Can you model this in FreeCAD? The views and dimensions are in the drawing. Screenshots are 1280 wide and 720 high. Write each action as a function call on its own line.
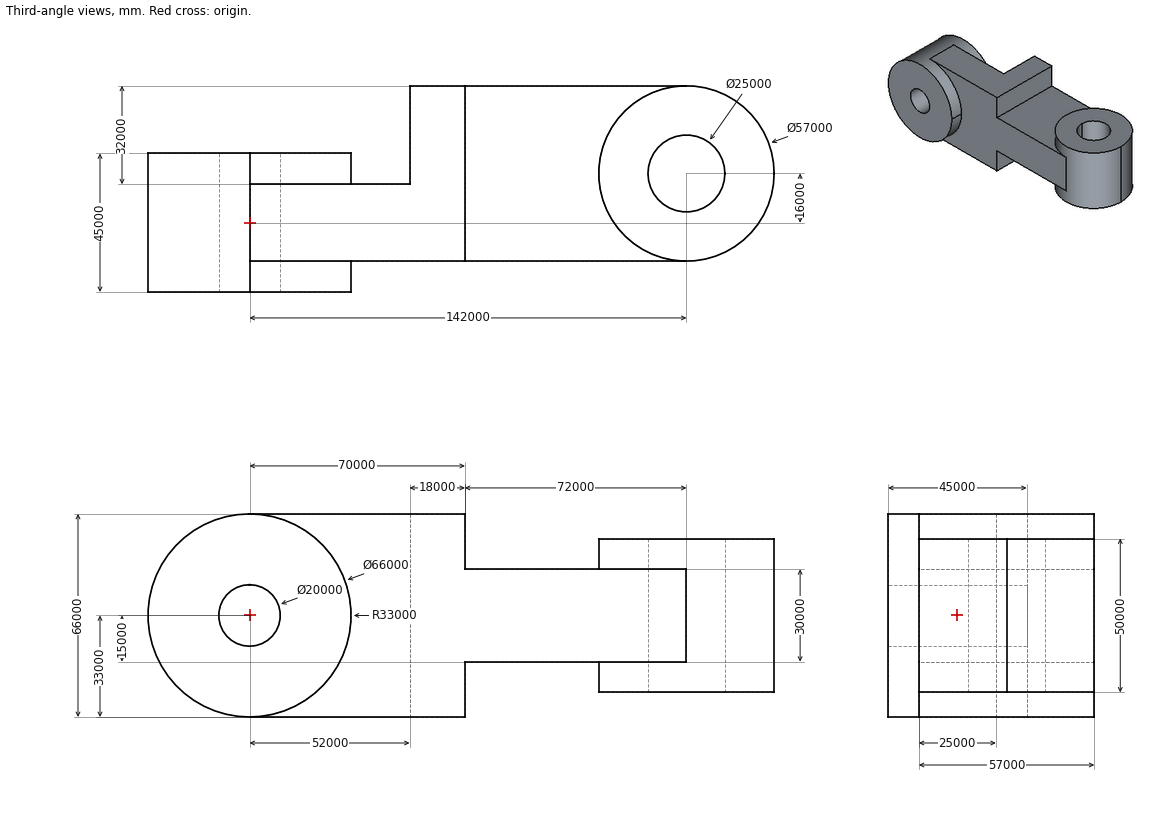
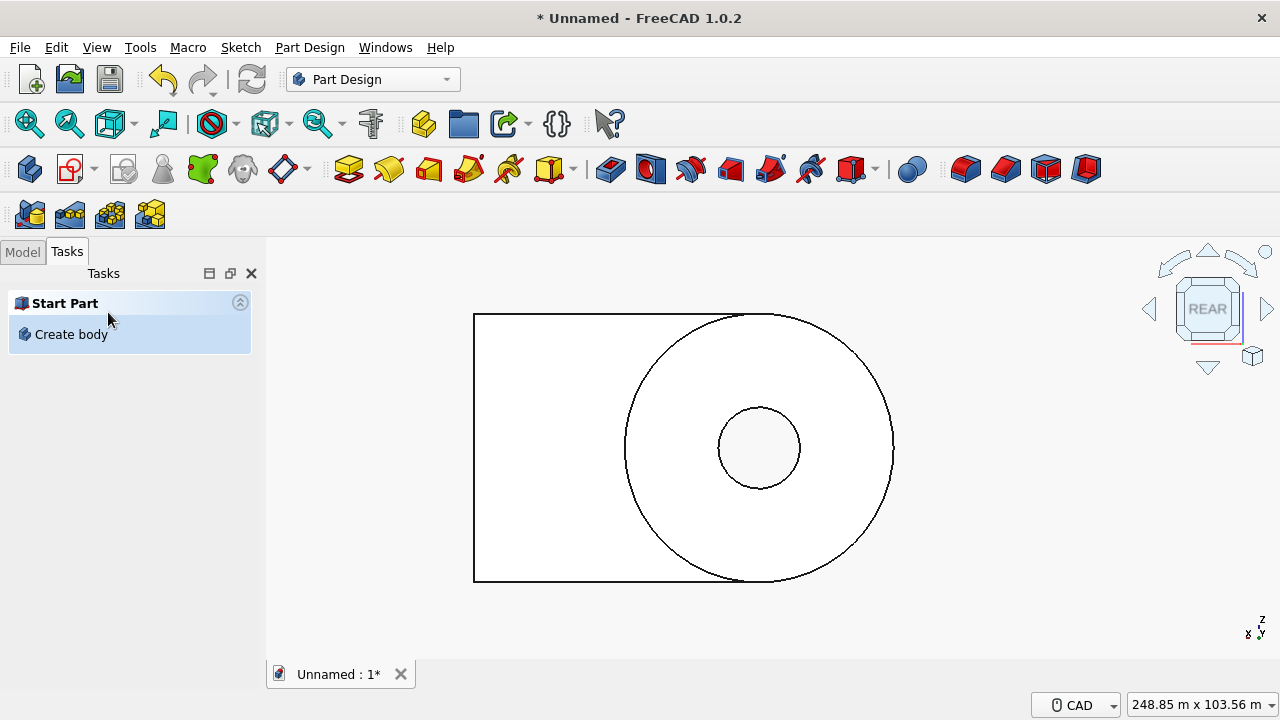
click(535, 409)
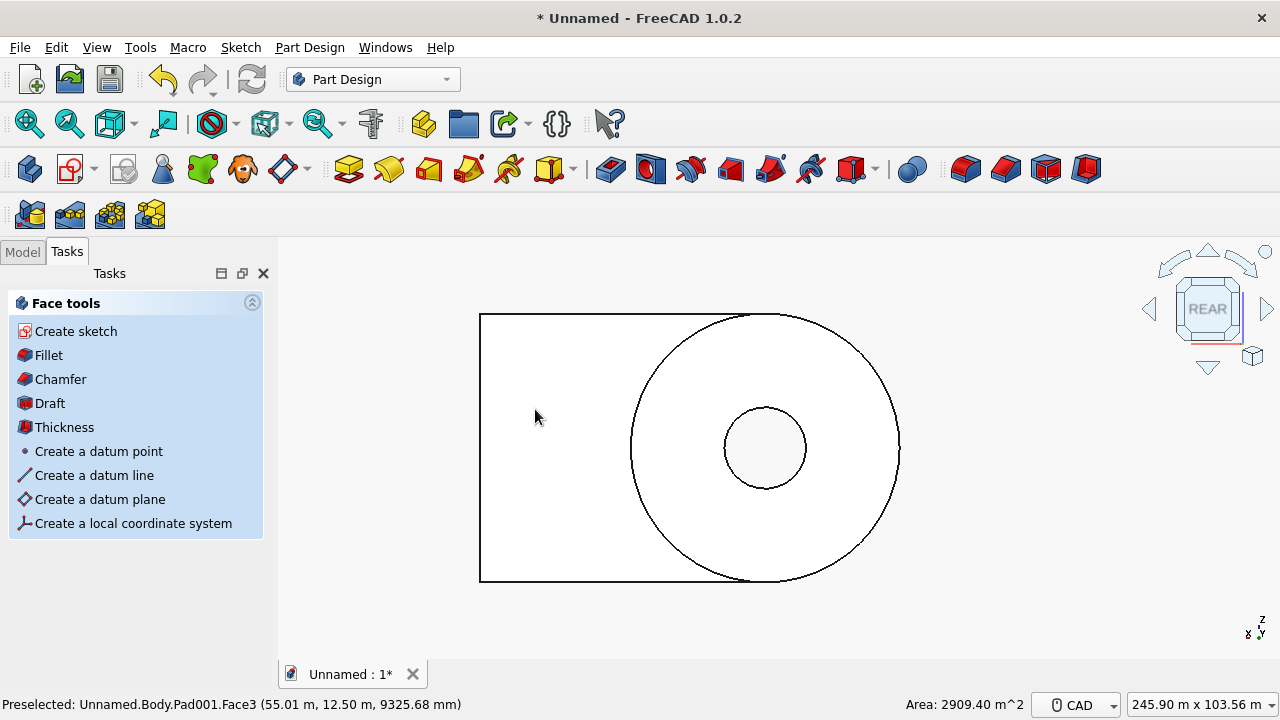
click(70, 170)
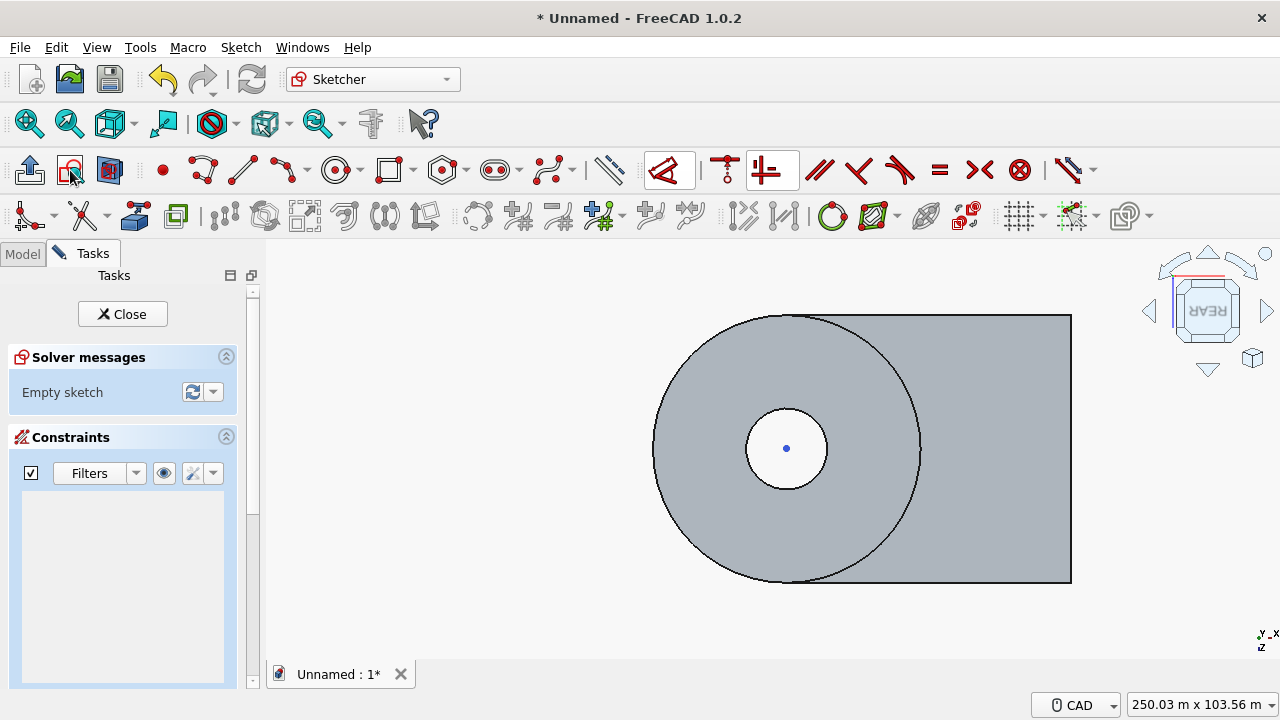
key(q)
key(s)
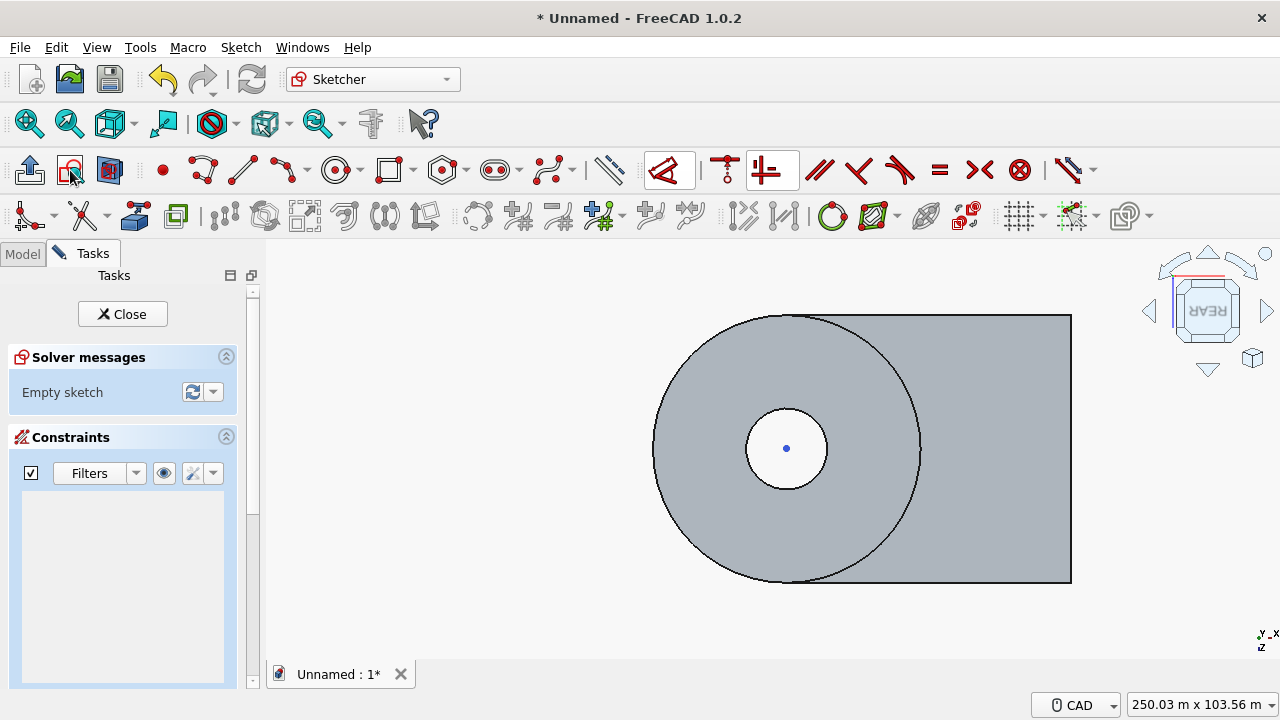
key(g)
key(r)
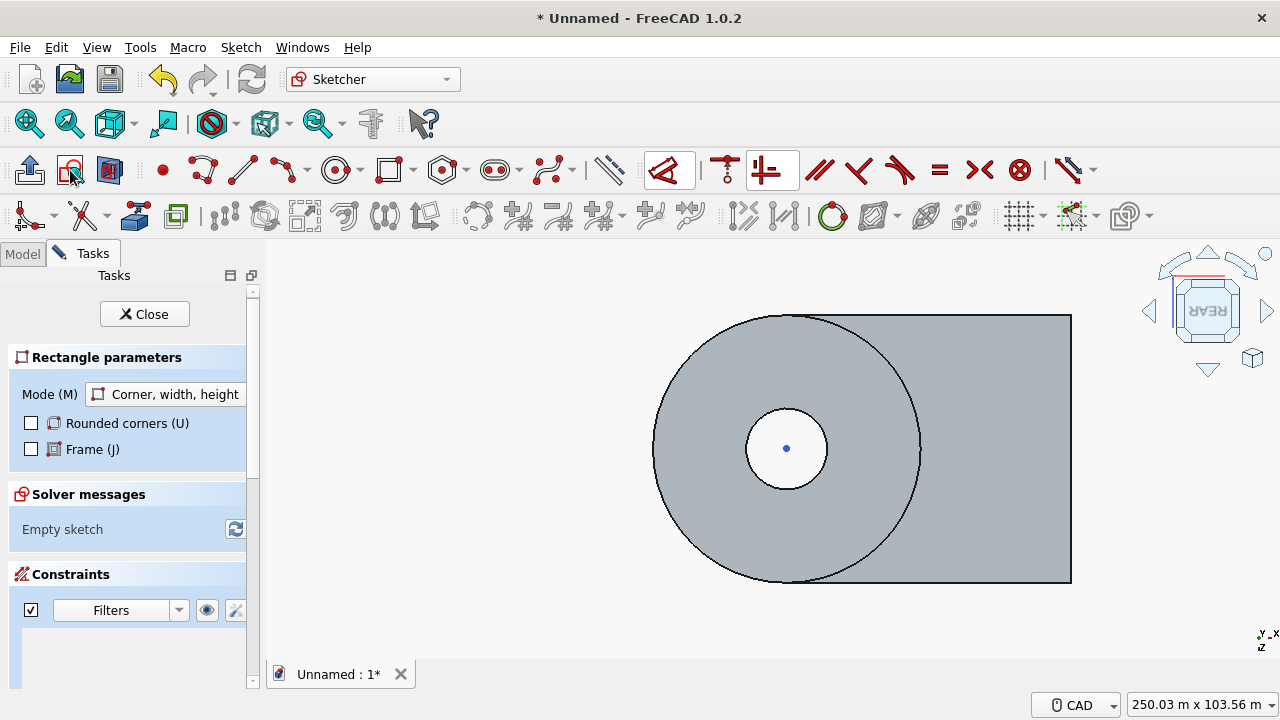
click(998, 315)
click(1071, 583)
key(Escape)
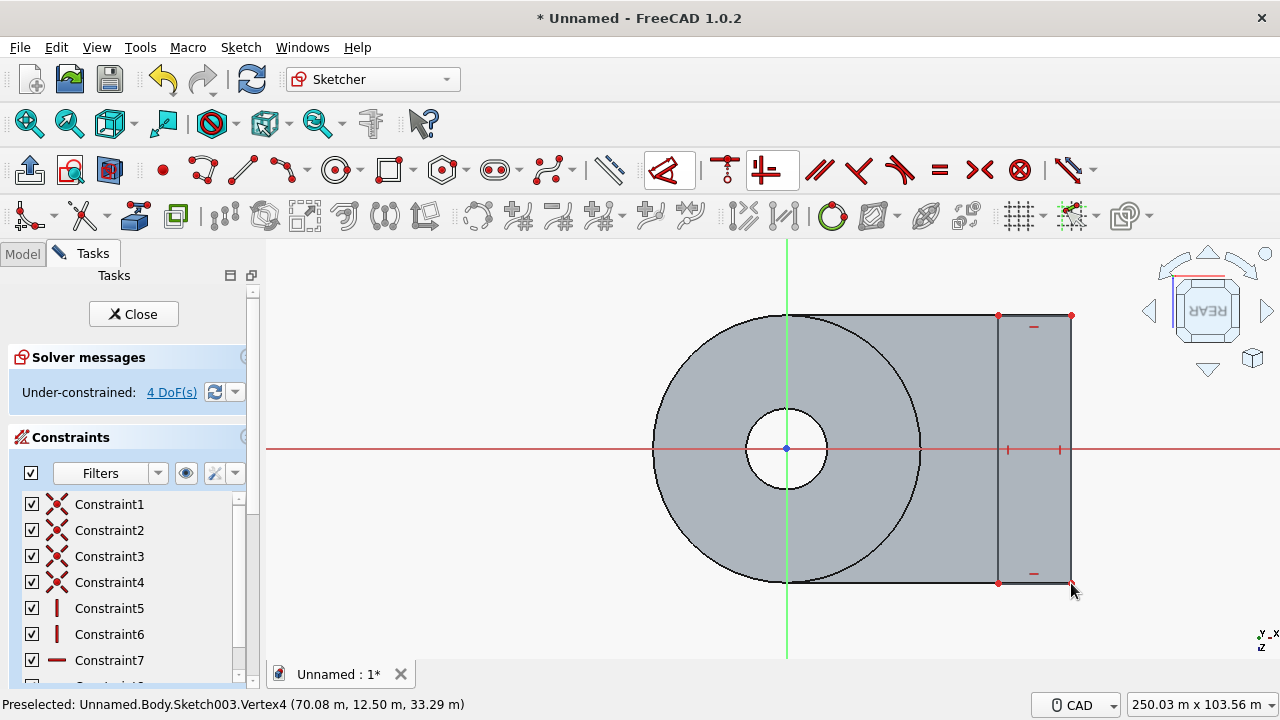
key(d)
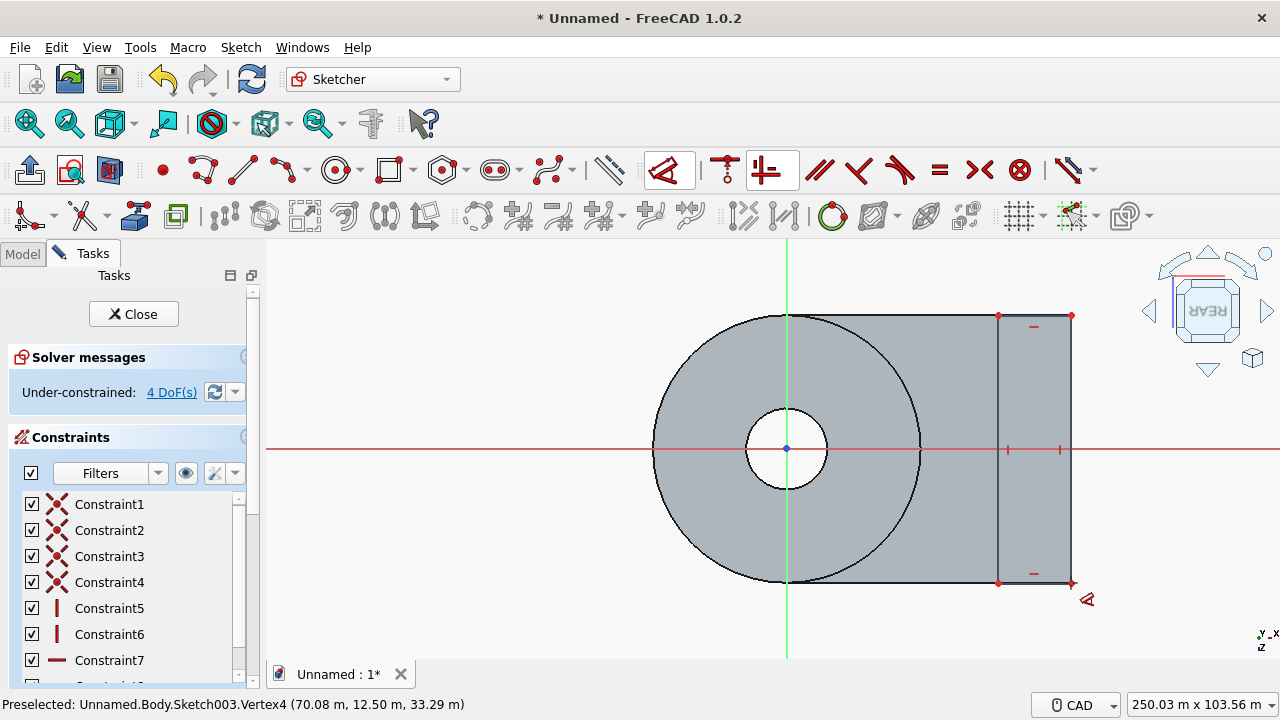
click(998, 396)
click(1032, 388)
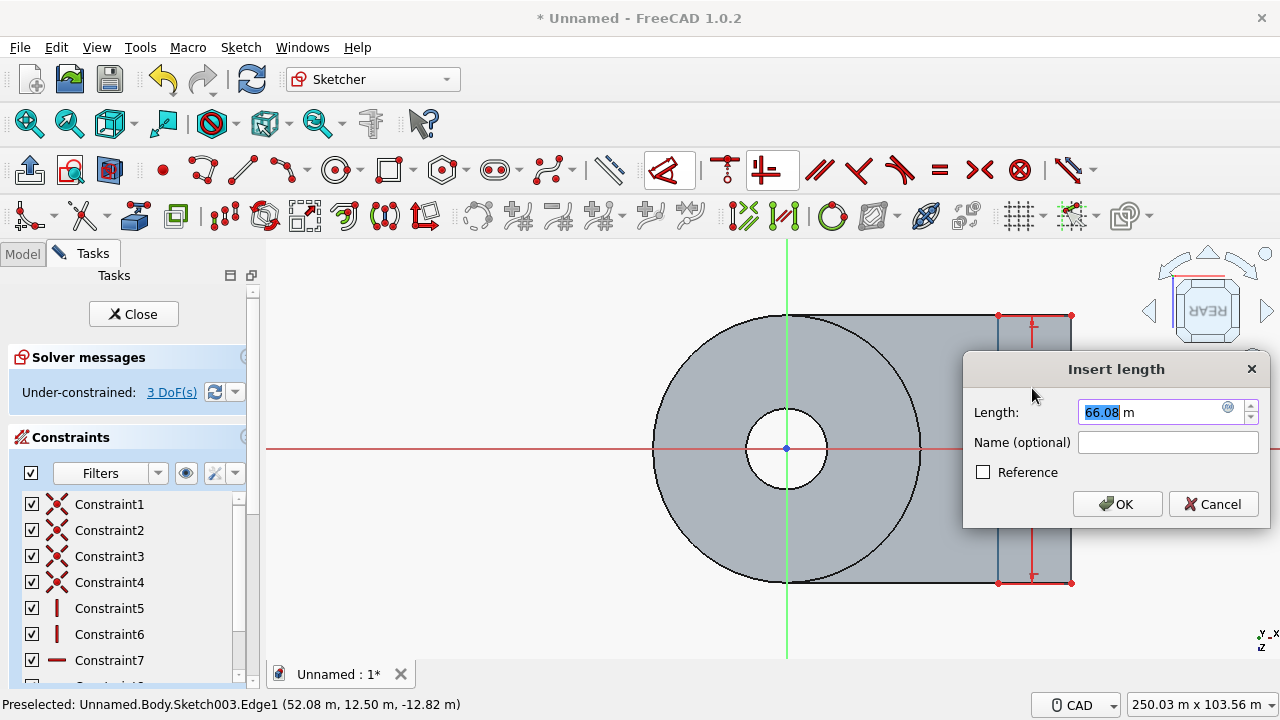
key(ctrl+a)
text(66000 mm)
key(Return)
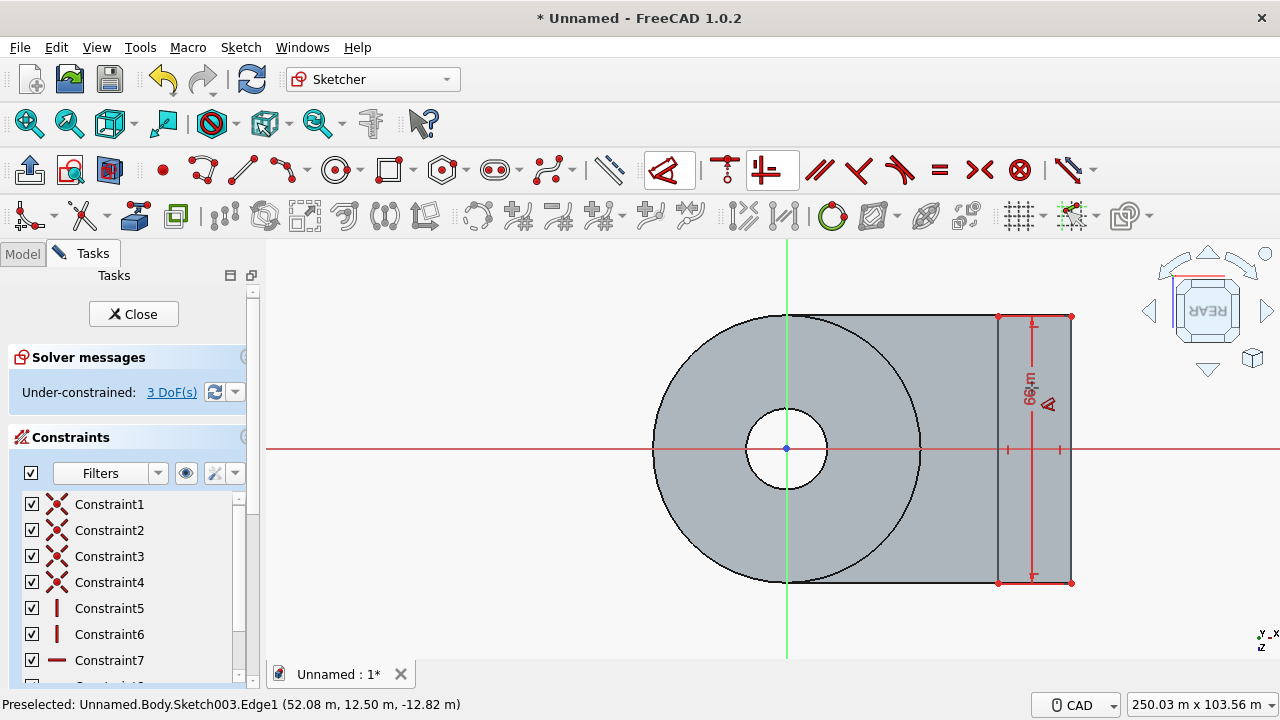
click(1020, 584)
click(1034, 618)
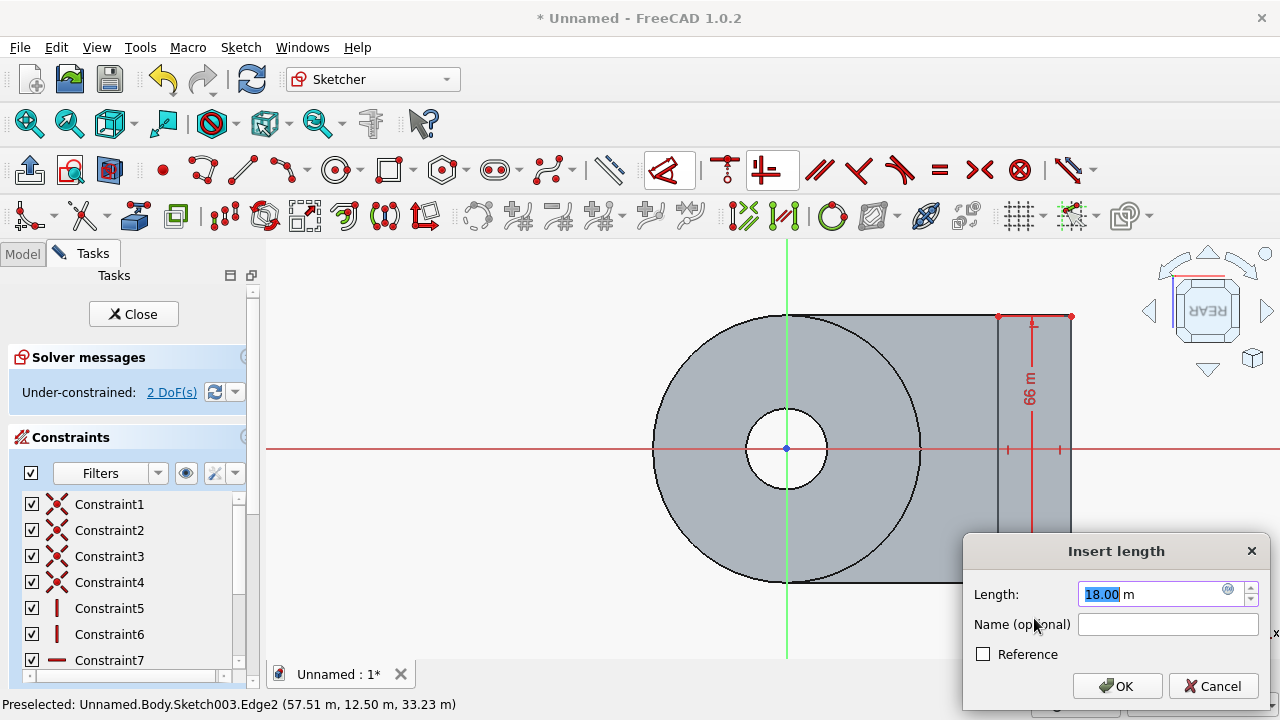
key(ctrl+a)
text(18000 mm)
key(Return)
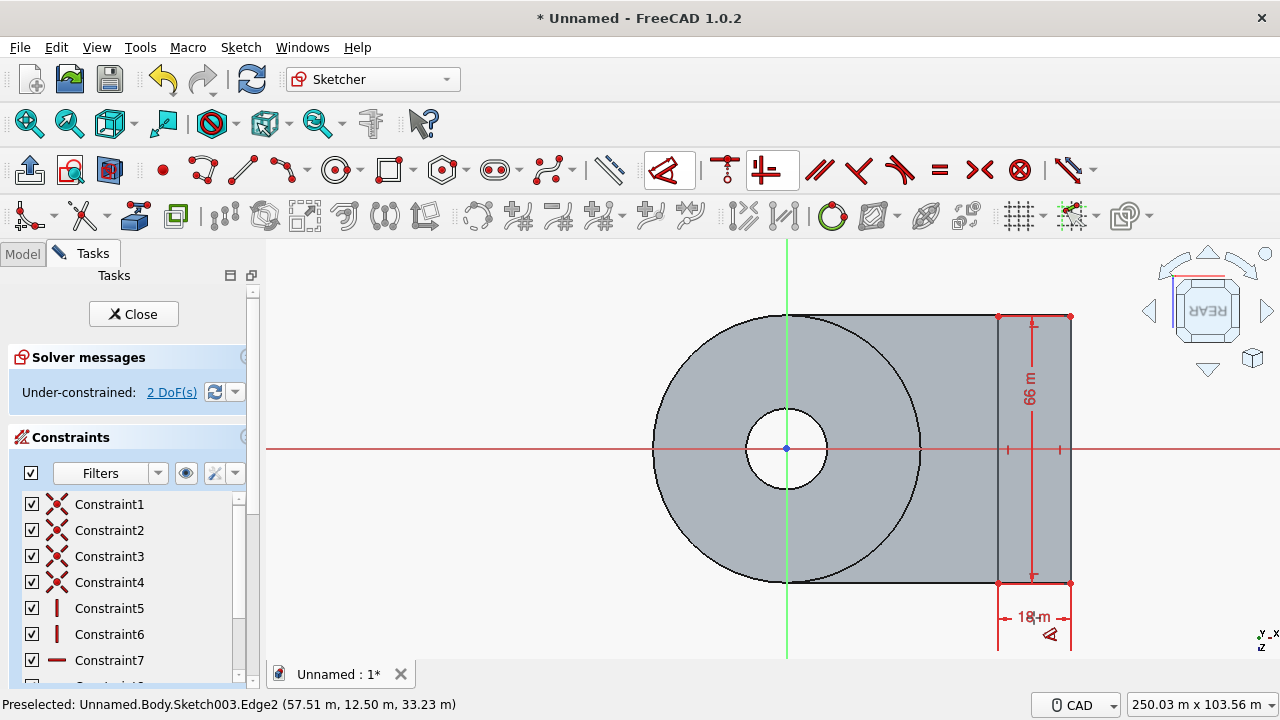
click(998, 316)
click(892, 282)